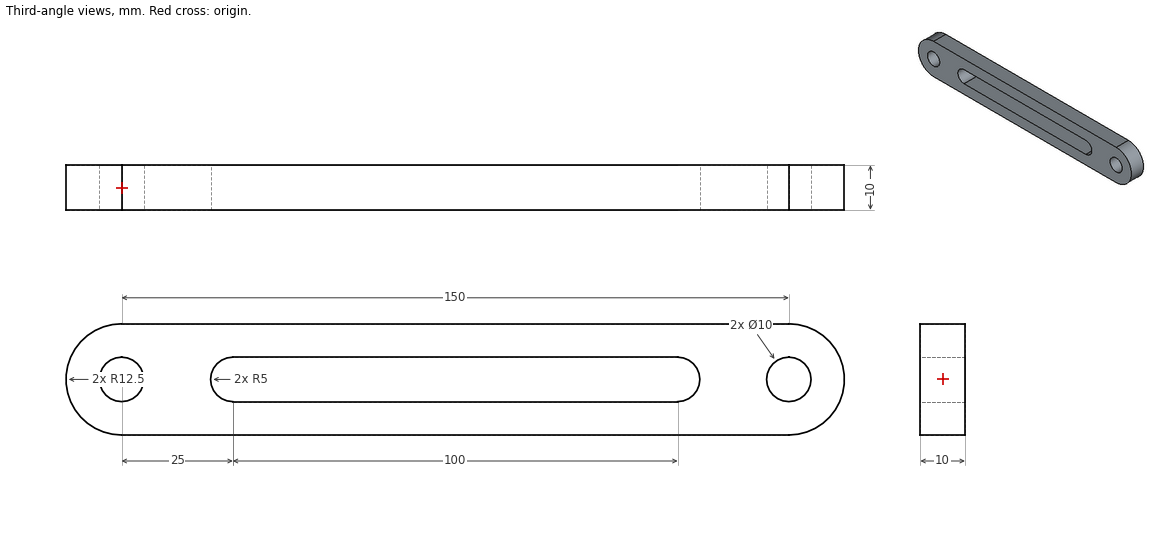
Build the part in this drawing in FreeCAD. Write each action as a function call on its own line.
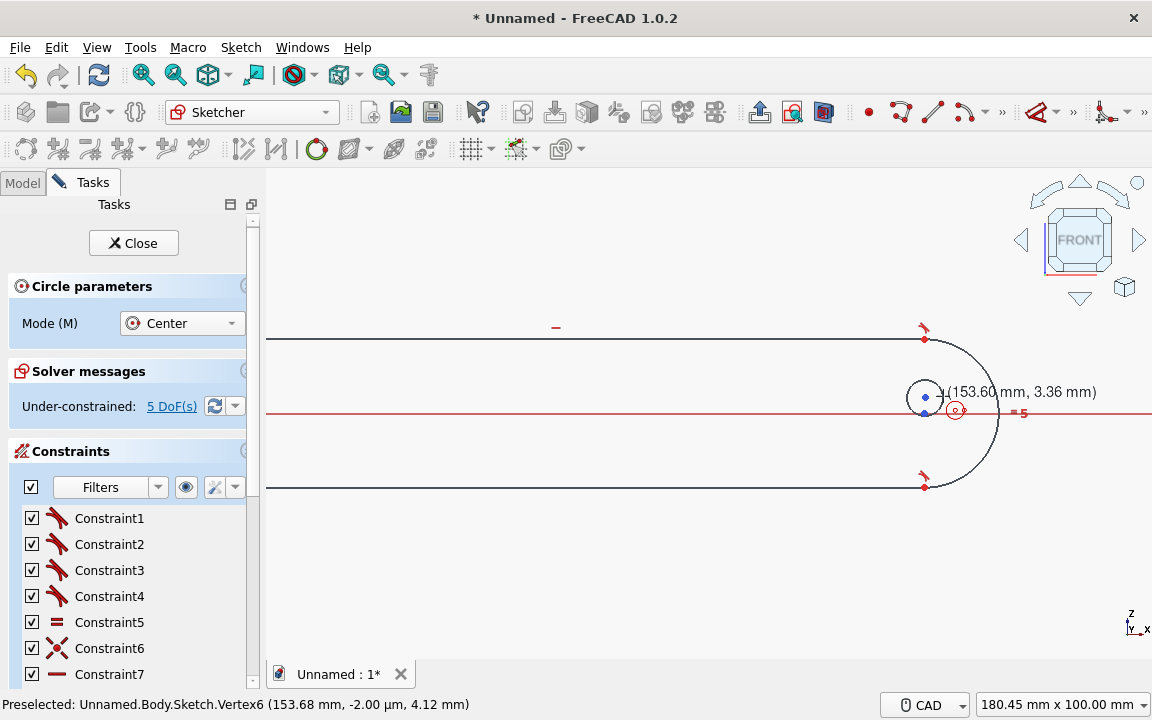
scroll(742, 413, down, 3)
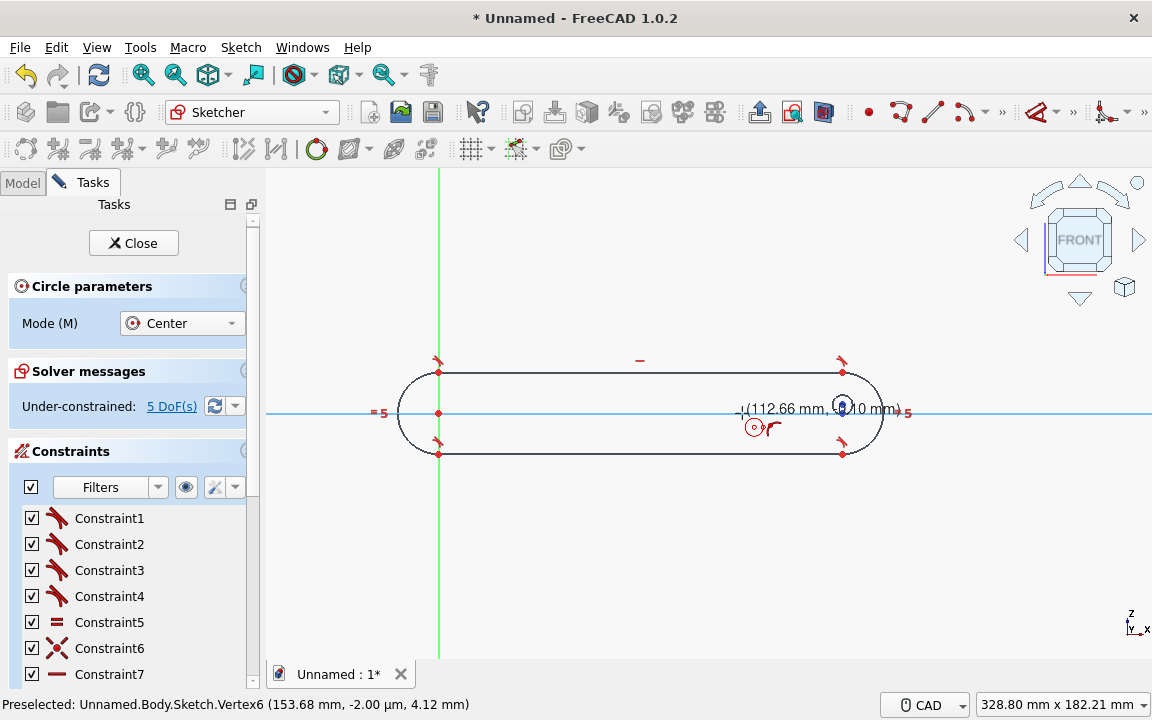
scroll(439, 414, up, 3)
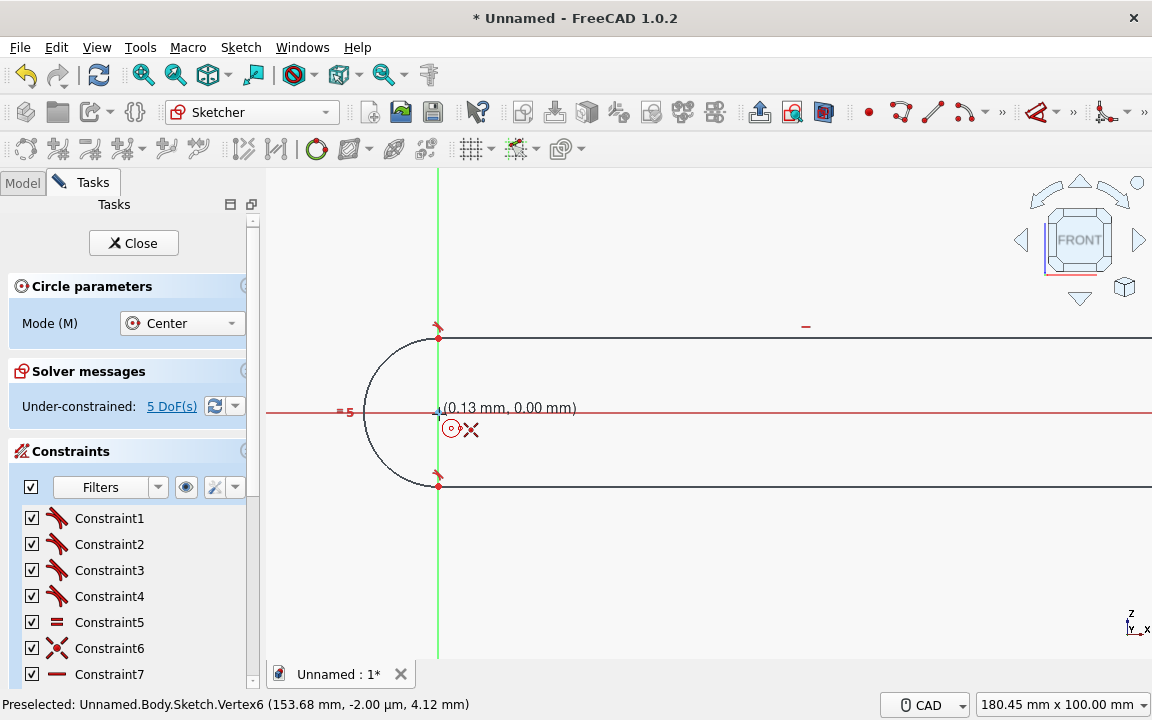
click(438, 413)
click(456, 395)
key(Escape)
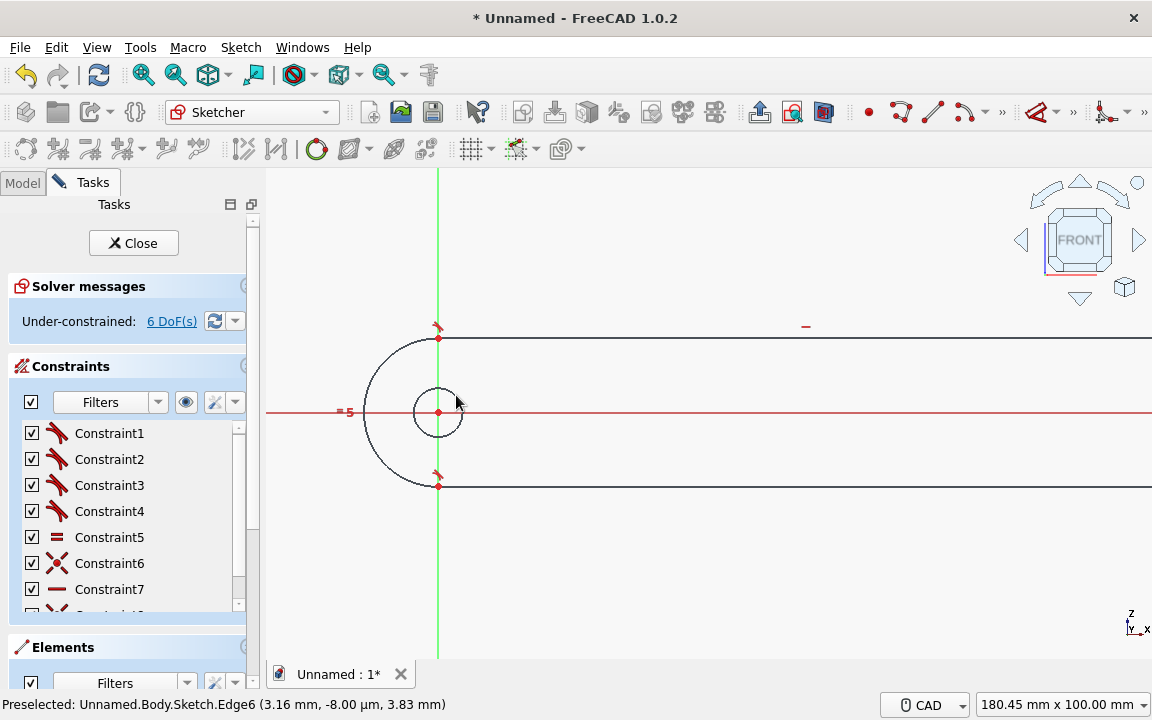
scroll(439, 415, down, 3)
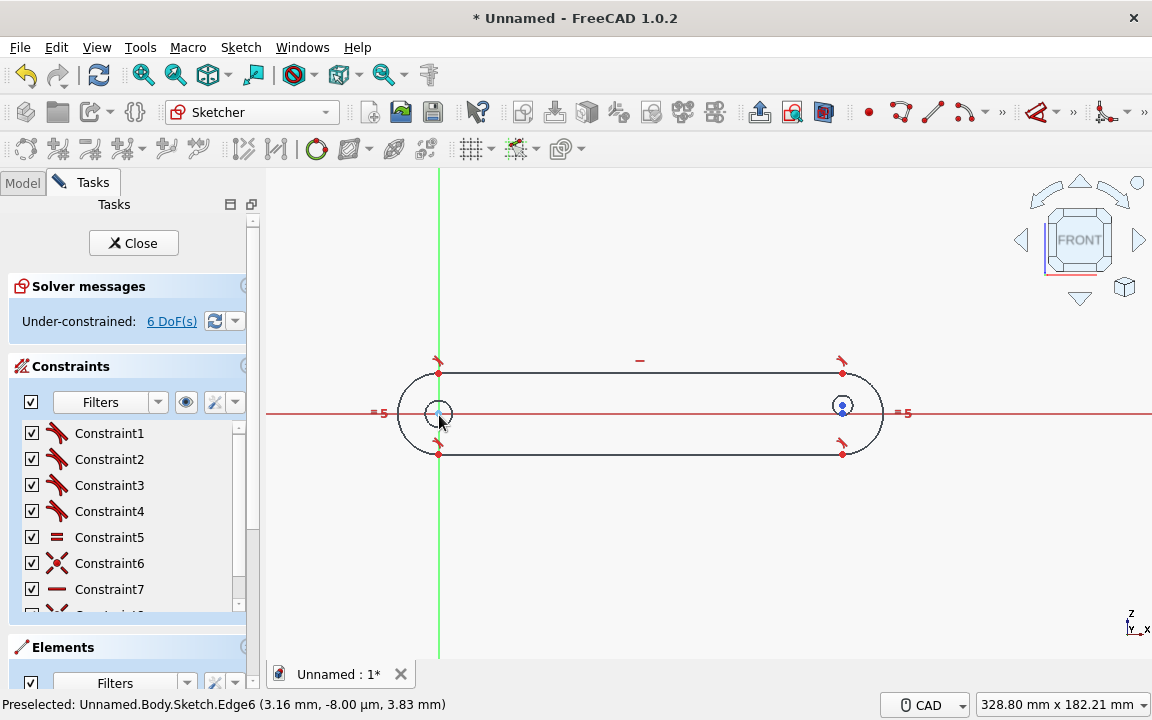
scroll(850, 398, up, 2)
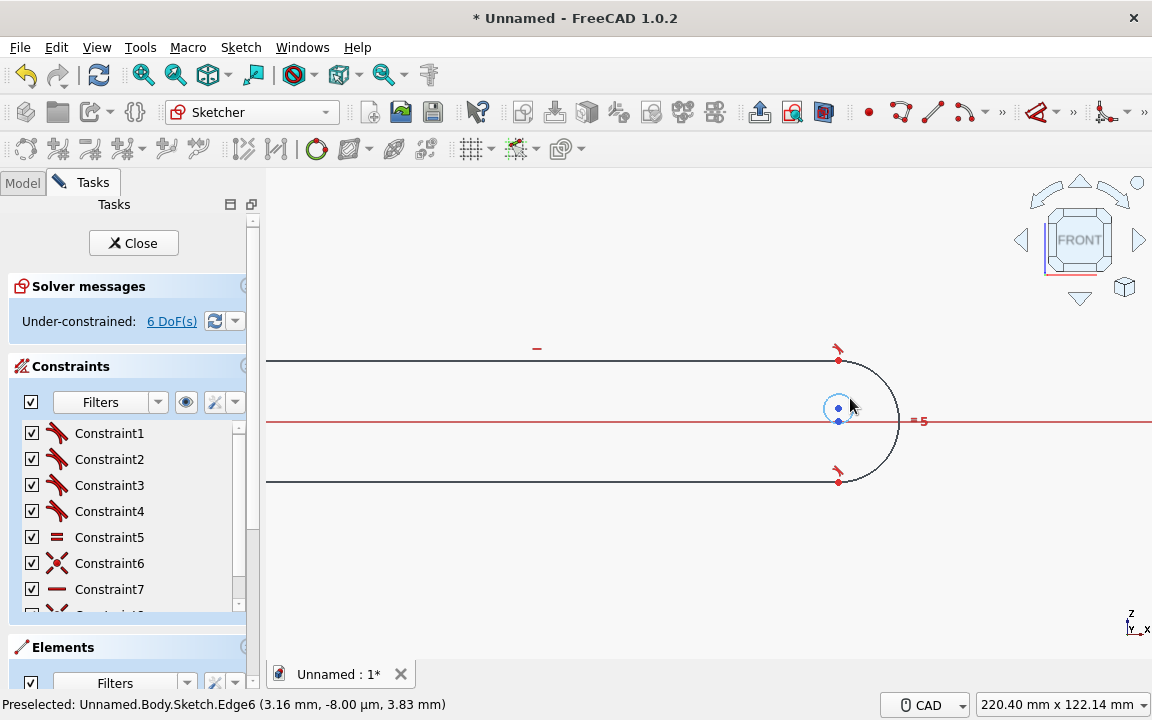
click(849, 398)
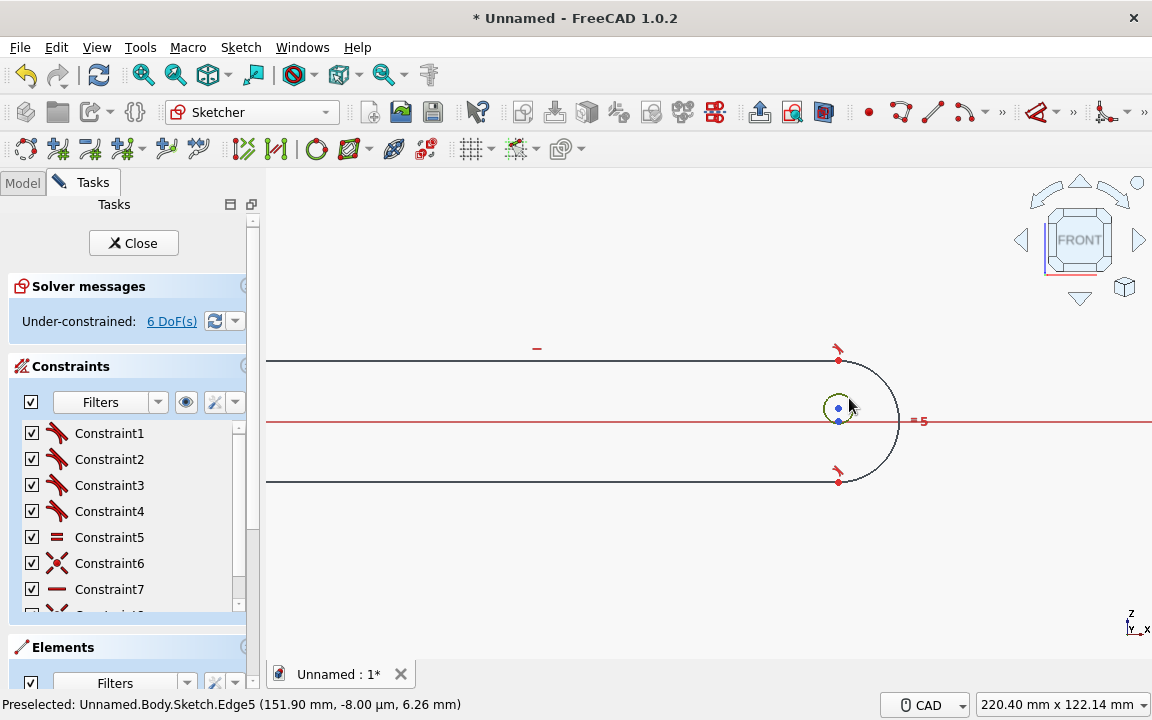
click(888, 457)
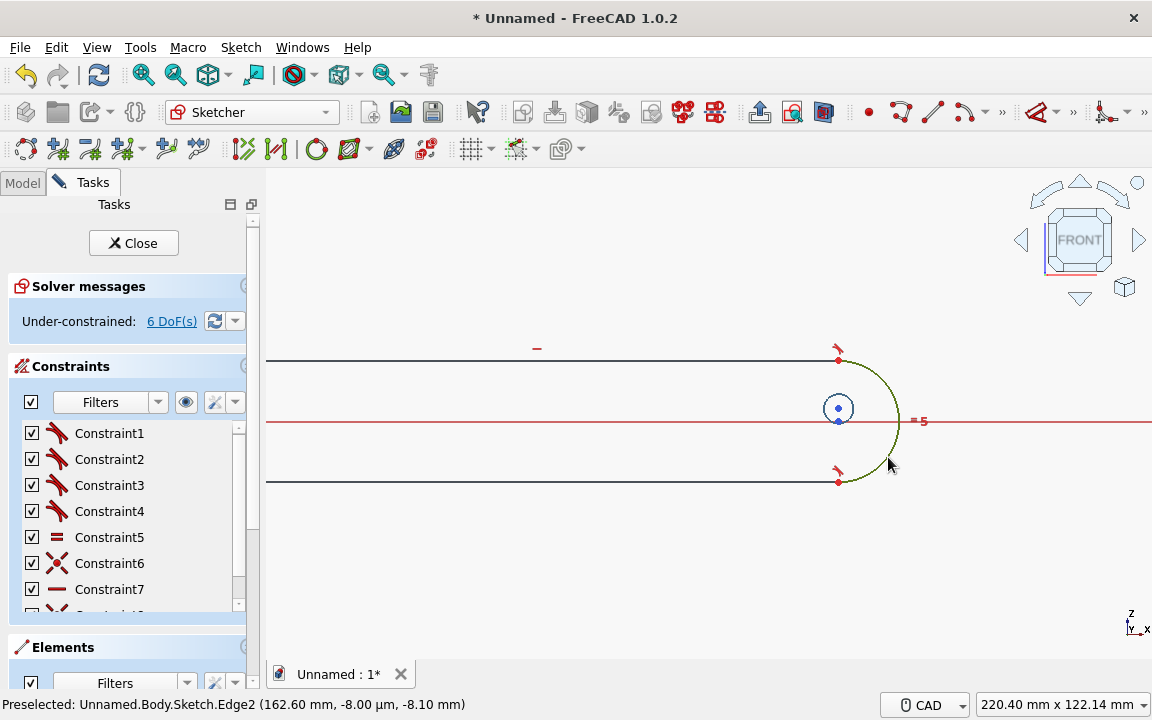
key(c)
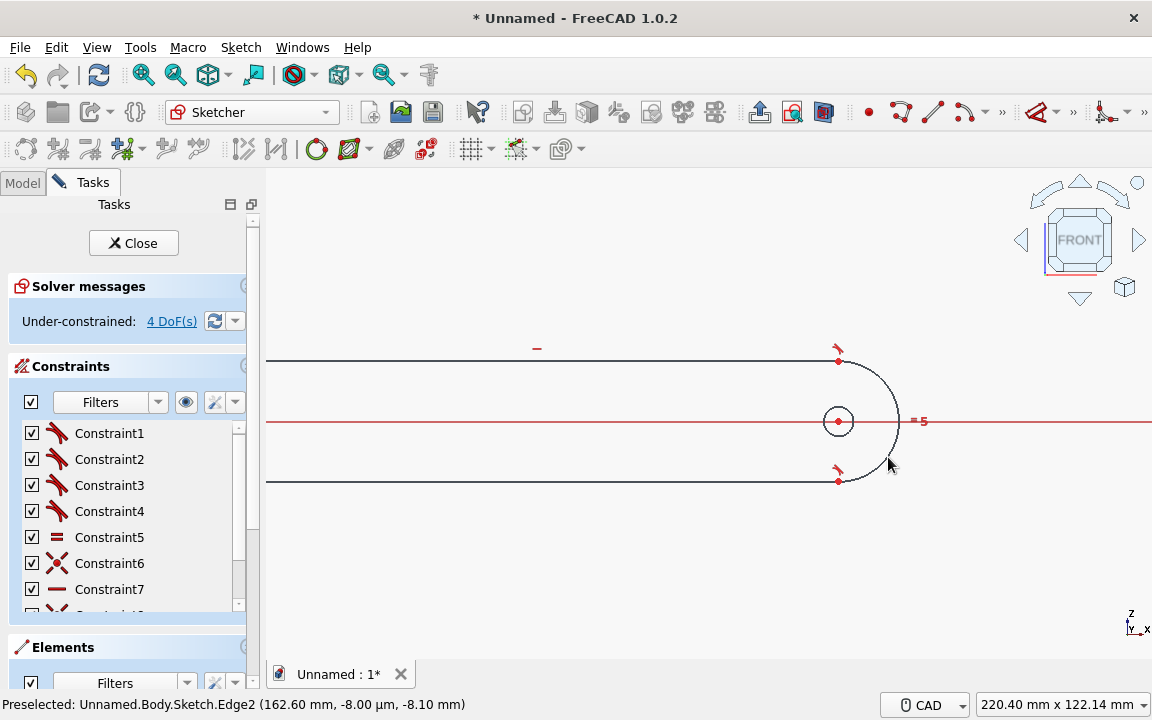
scroll(849, 411, up, 2)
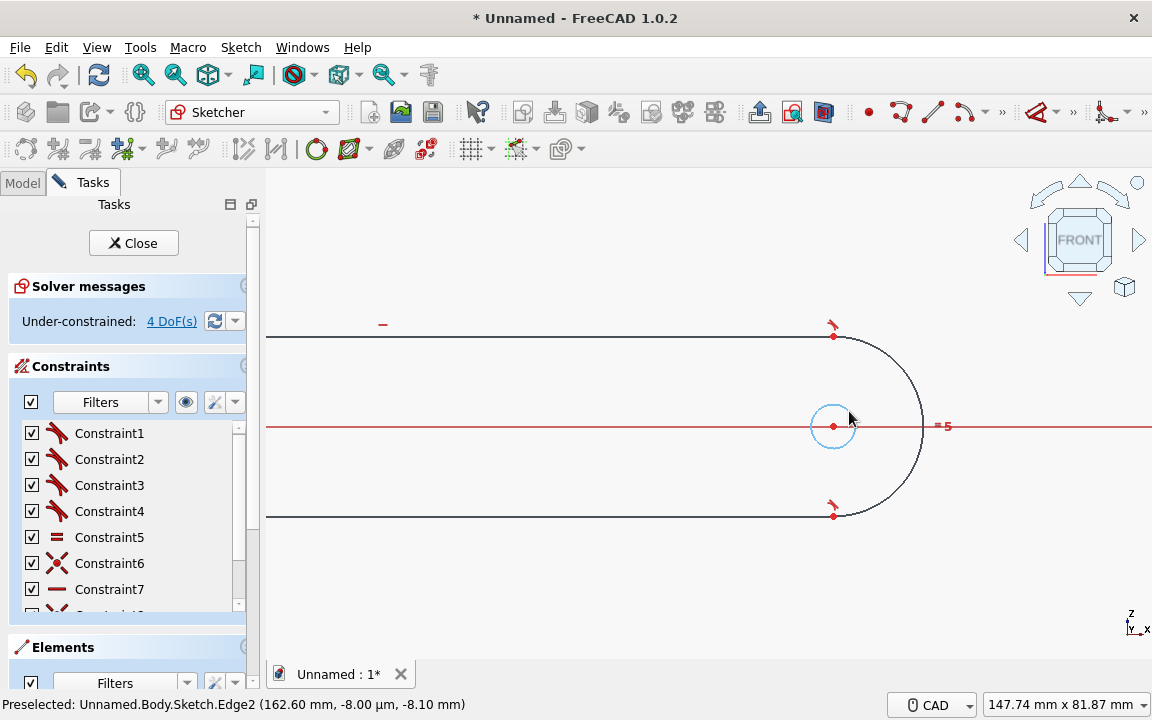
click(849, 411)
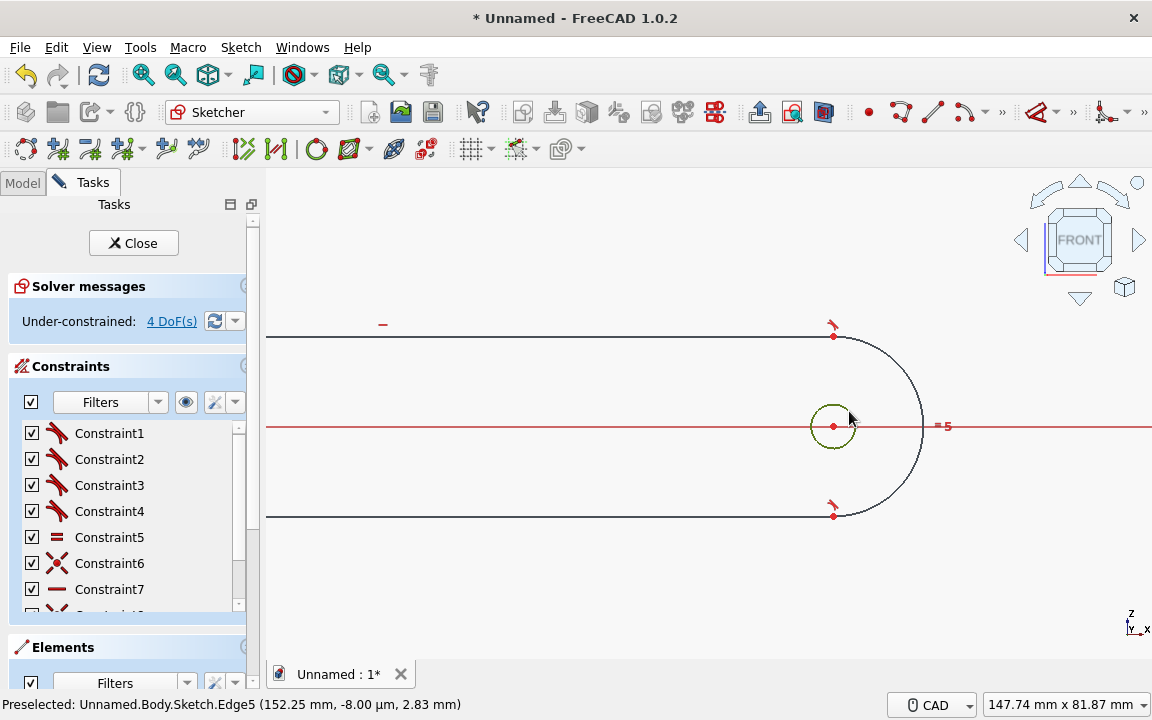
scroll(850, 403, down, 4)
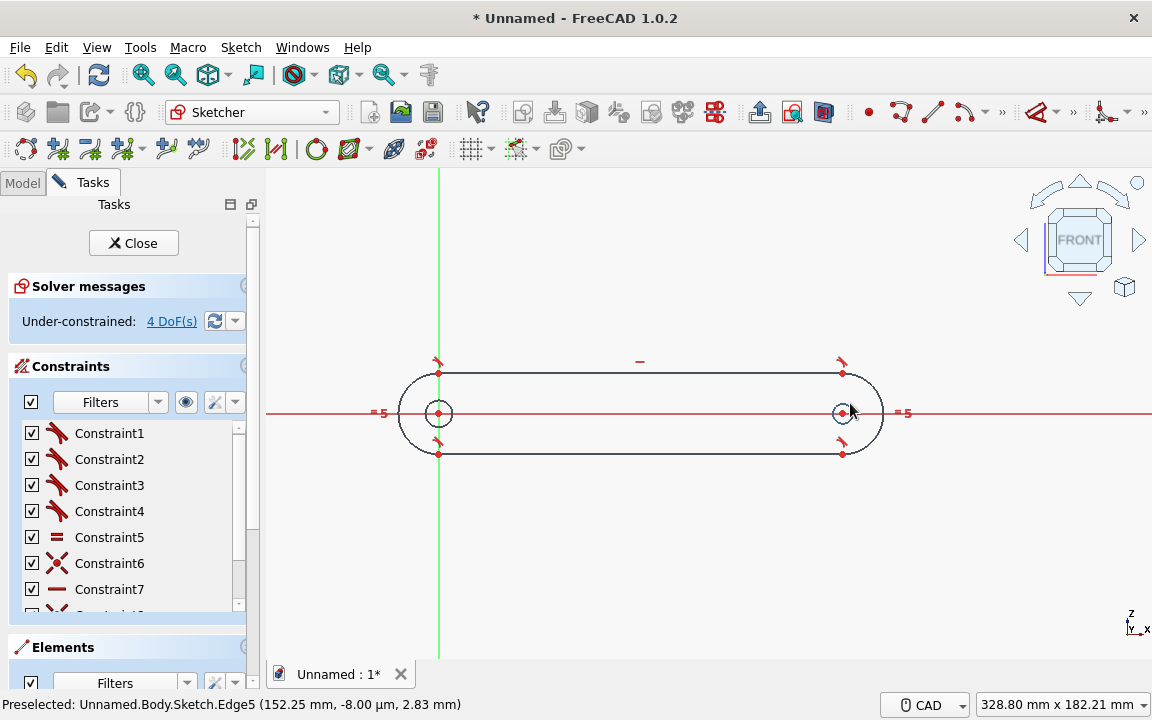
scroll(448, 404, up, 2)